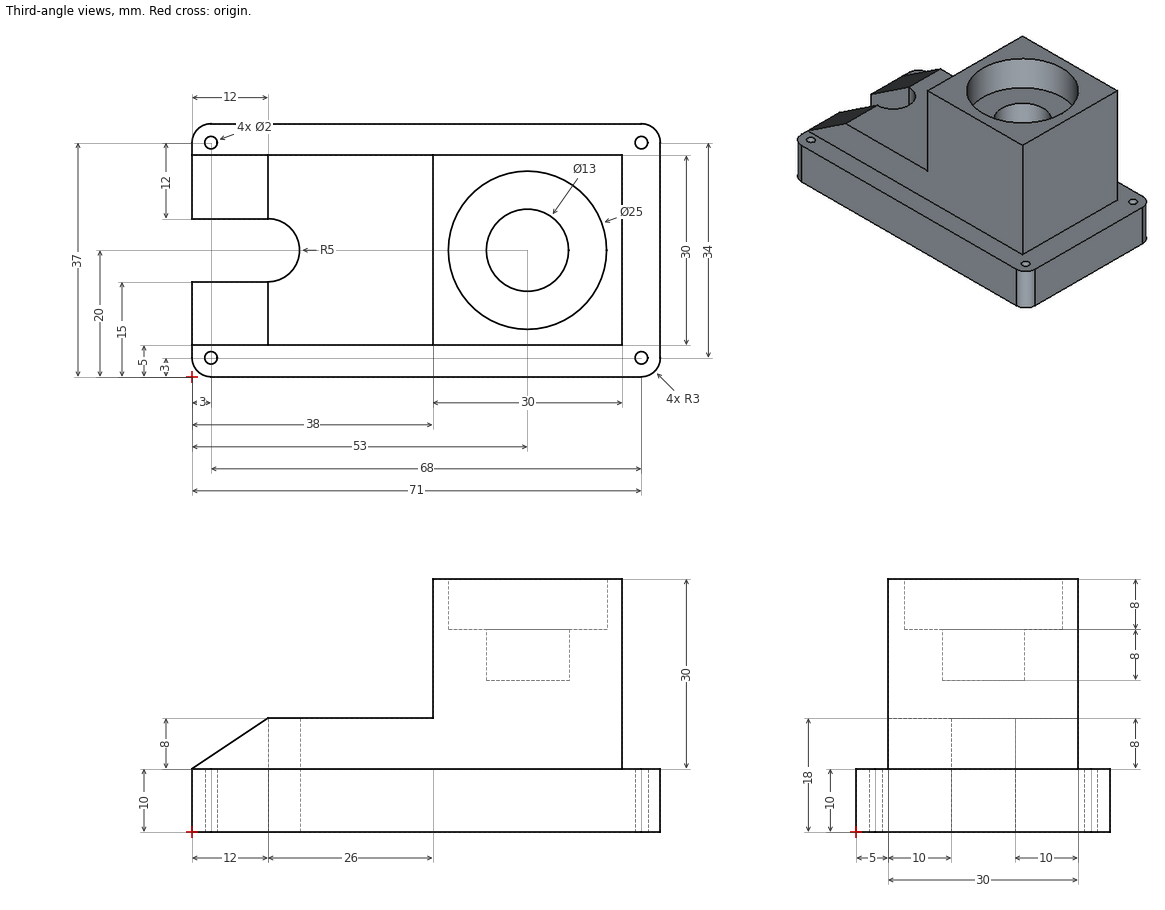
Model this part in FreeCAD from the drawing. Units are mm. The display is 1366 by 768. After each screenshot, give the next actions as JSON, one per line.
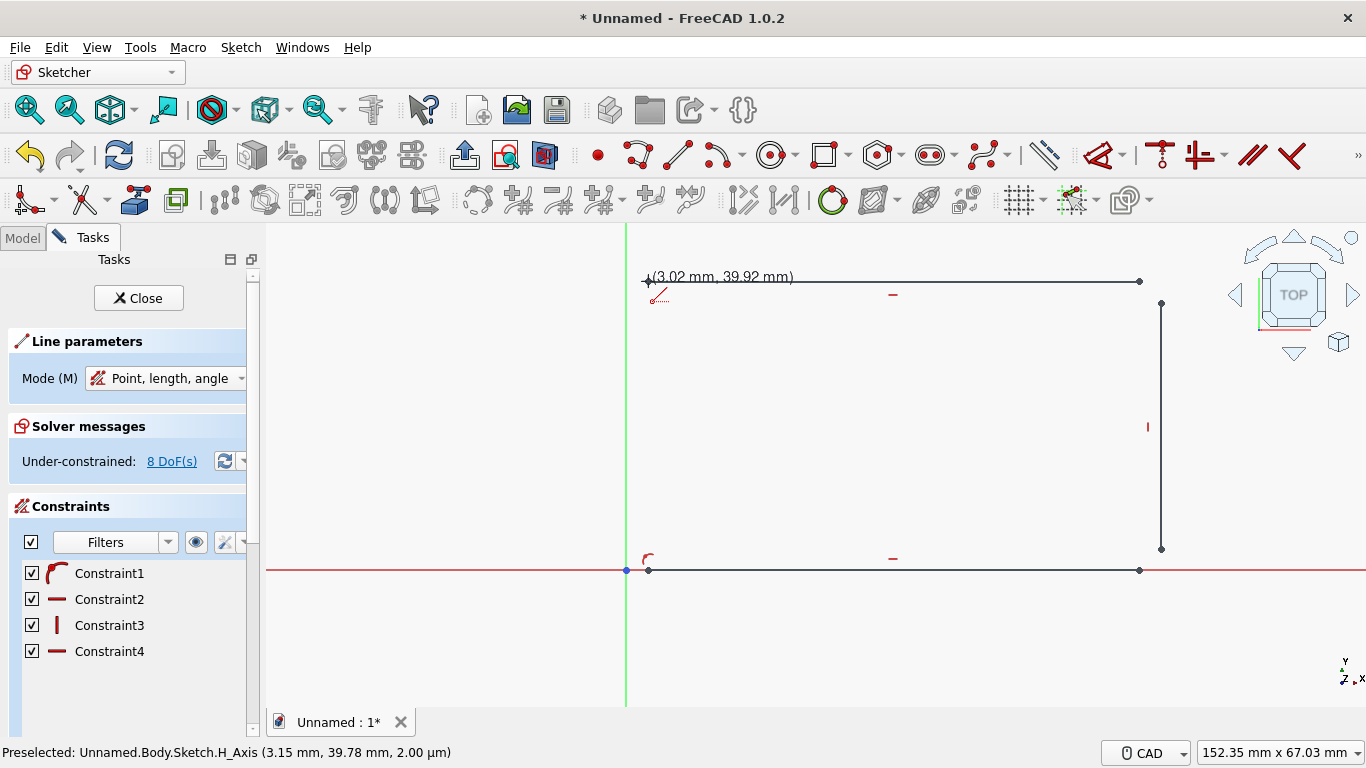
{"action": "key", "text": "g m"}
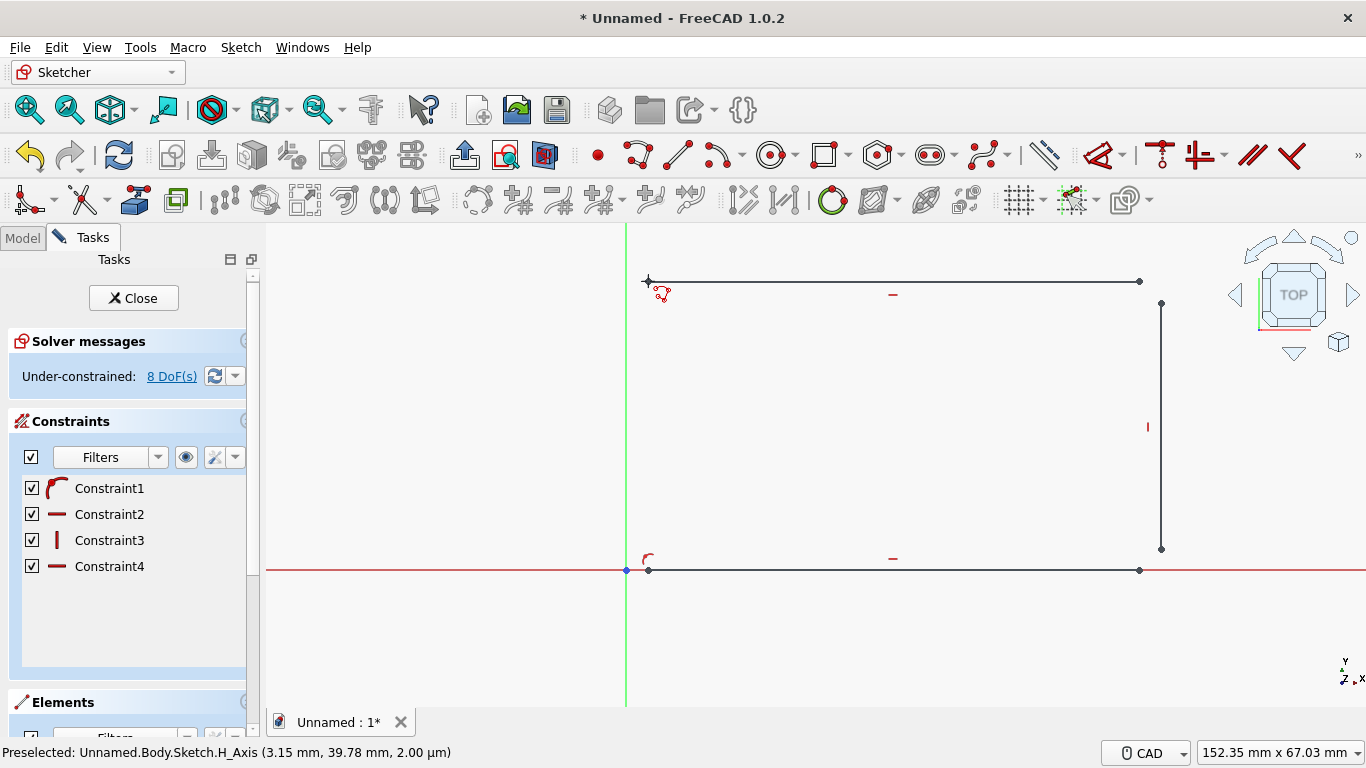
{"action": "left_click", "coordinate": [626, 303]}
{"action": "left_click", "coordinate": [635, 390]}
{"action": "left_click", "coordinate": [713, 390]}
{"action": "right_click", "coordinate": [713, 390]}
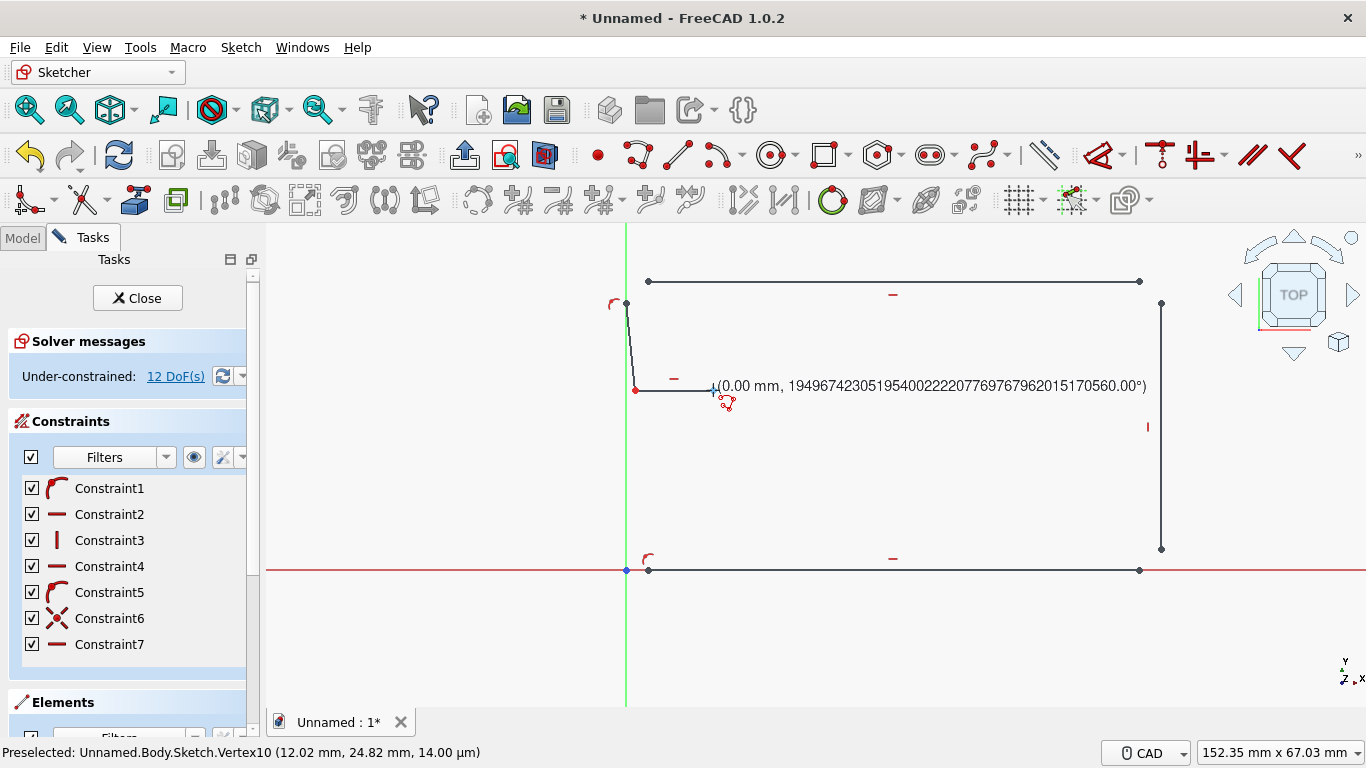
{"action": "left_click", "coordinate": [713, 462]}
{"action": "left_click", "coordinate": [626, 462]}
{"action": "left_click", "coordinate": [635, 549]}
{"action": "right_click", "coordinate": [635, 549]}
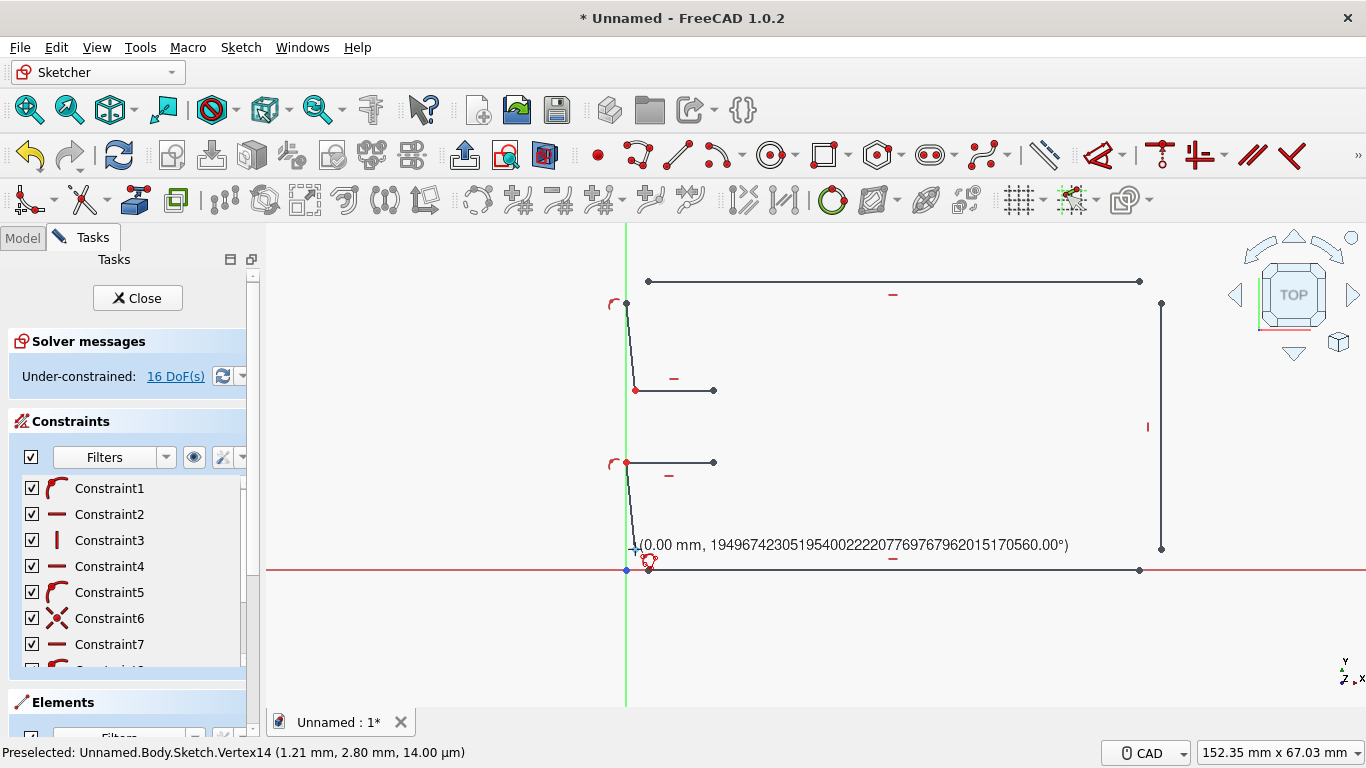
{"action": "key", "text": "g 3 a"}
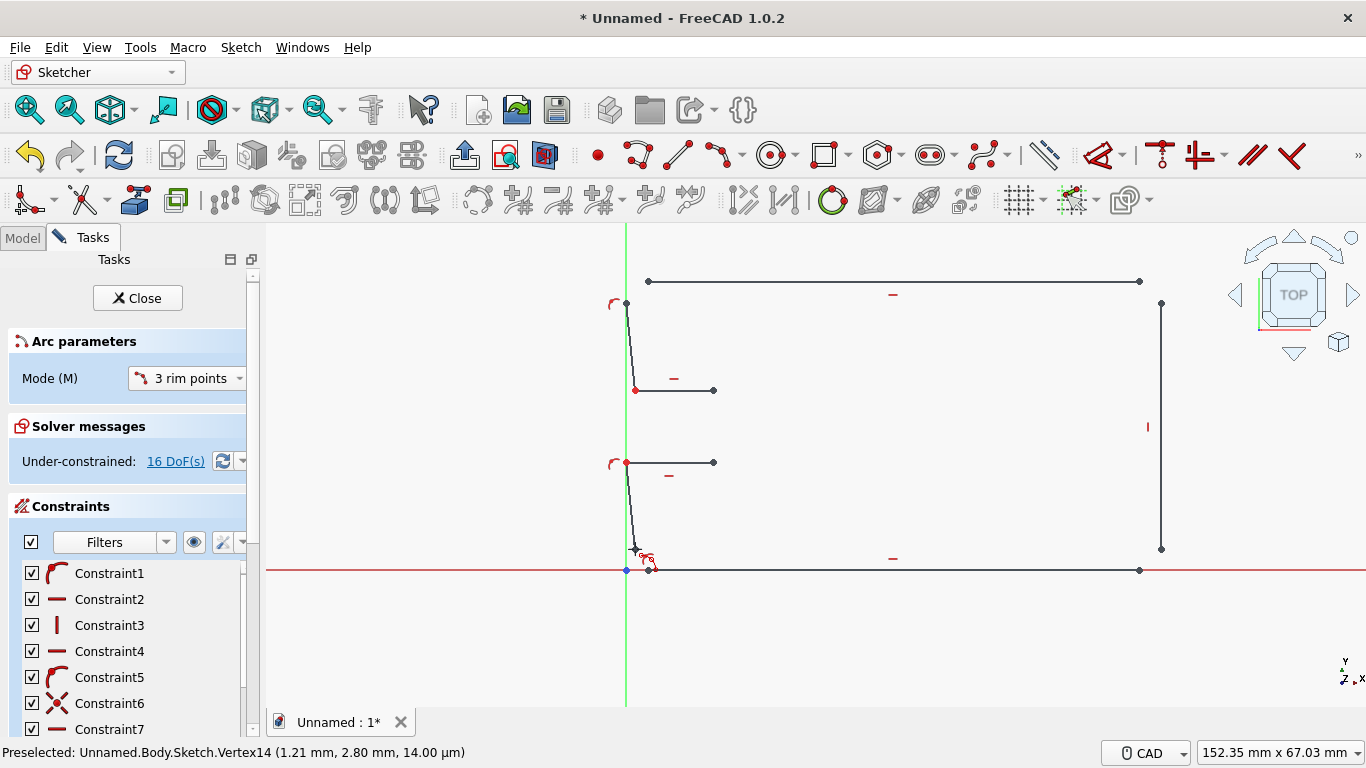
{"action": "left_click", "coordinate": [1139, 561]}
{"action": "left_click", "coordinate": [1161, 550]}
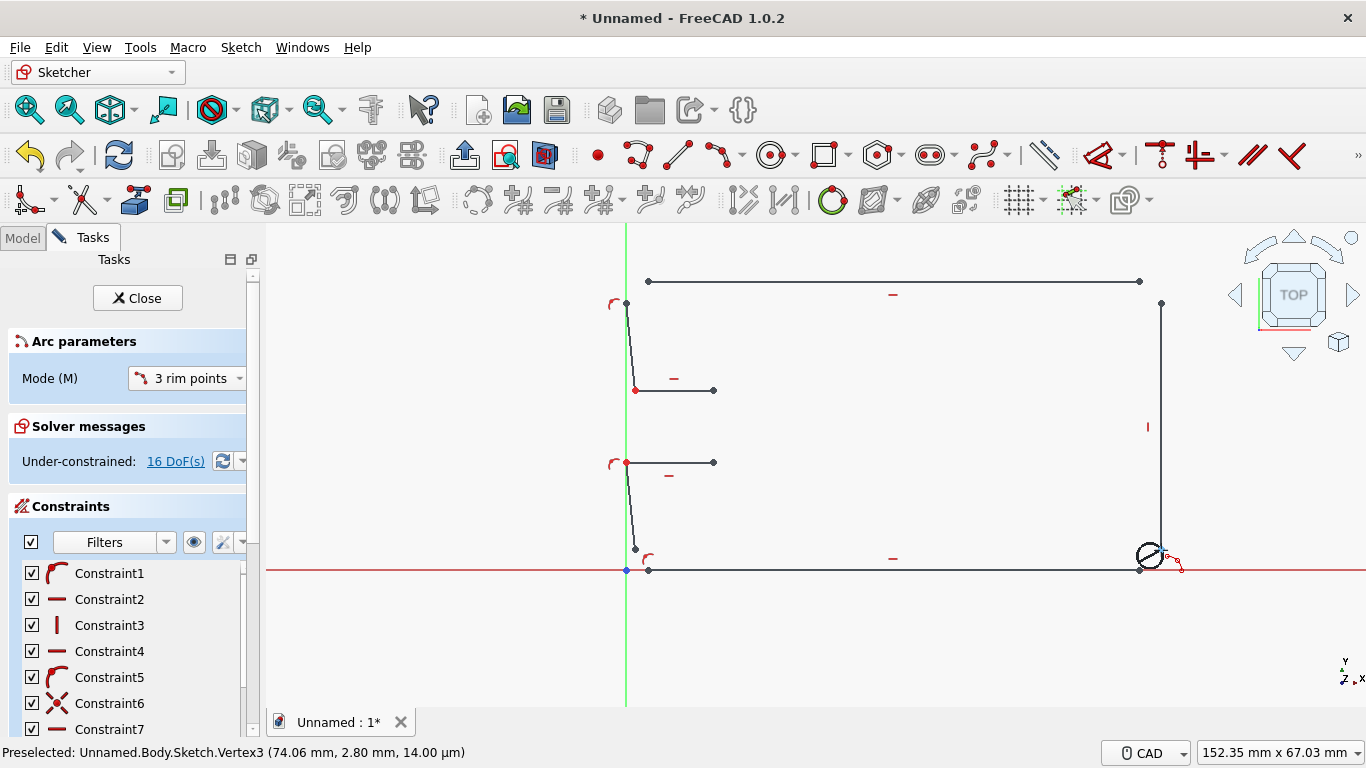
{"action": "scroll", "coordinate": [1154, 564], "scroll_direction": "up", "scroll_amount": 5}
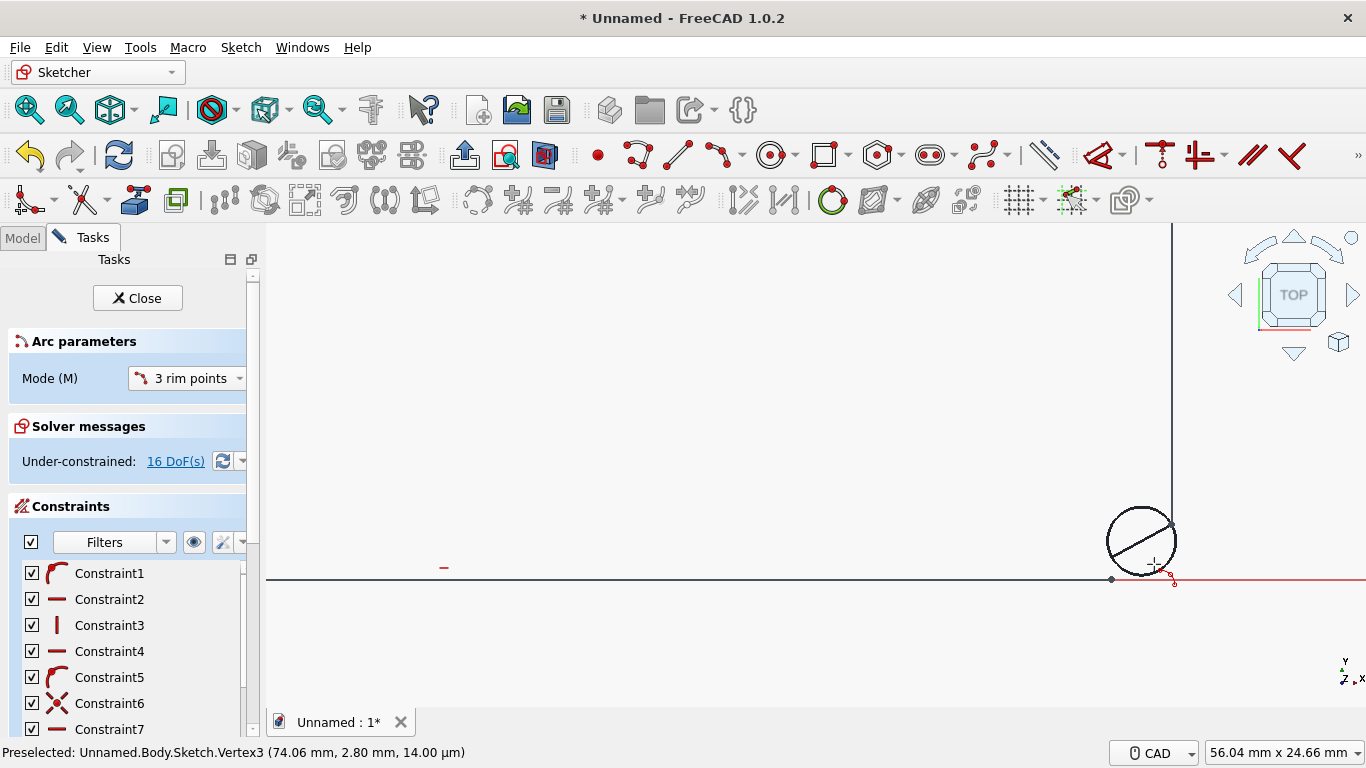
{"action": "left_click", "coordinate": [1153, 562]}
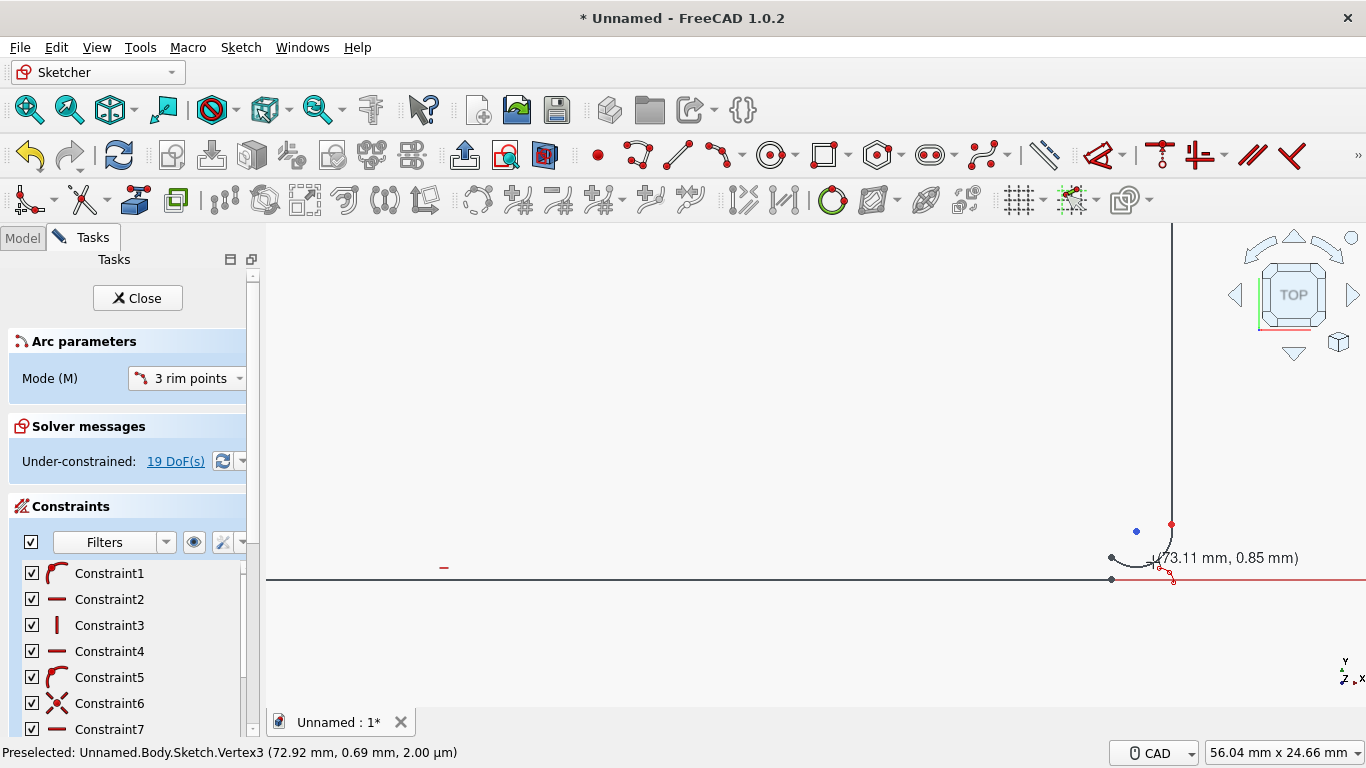
{"action": "scroll", "coordinate": [924, 627], "scroll_direction": "down", "scroll_amount": 5}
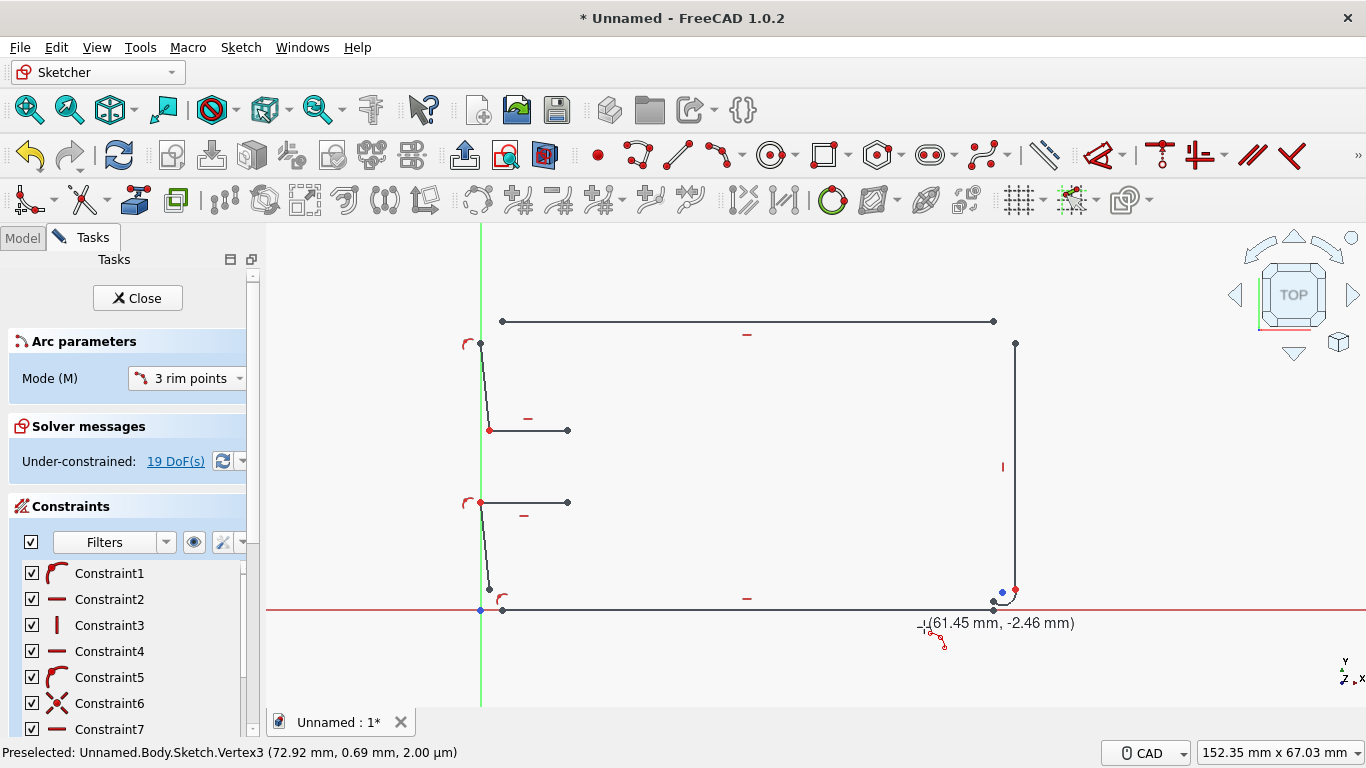
{"action": "left_click", "coordinate": [1015, 344]}
{"action": "left_click", "coordinate": [993, 322]}